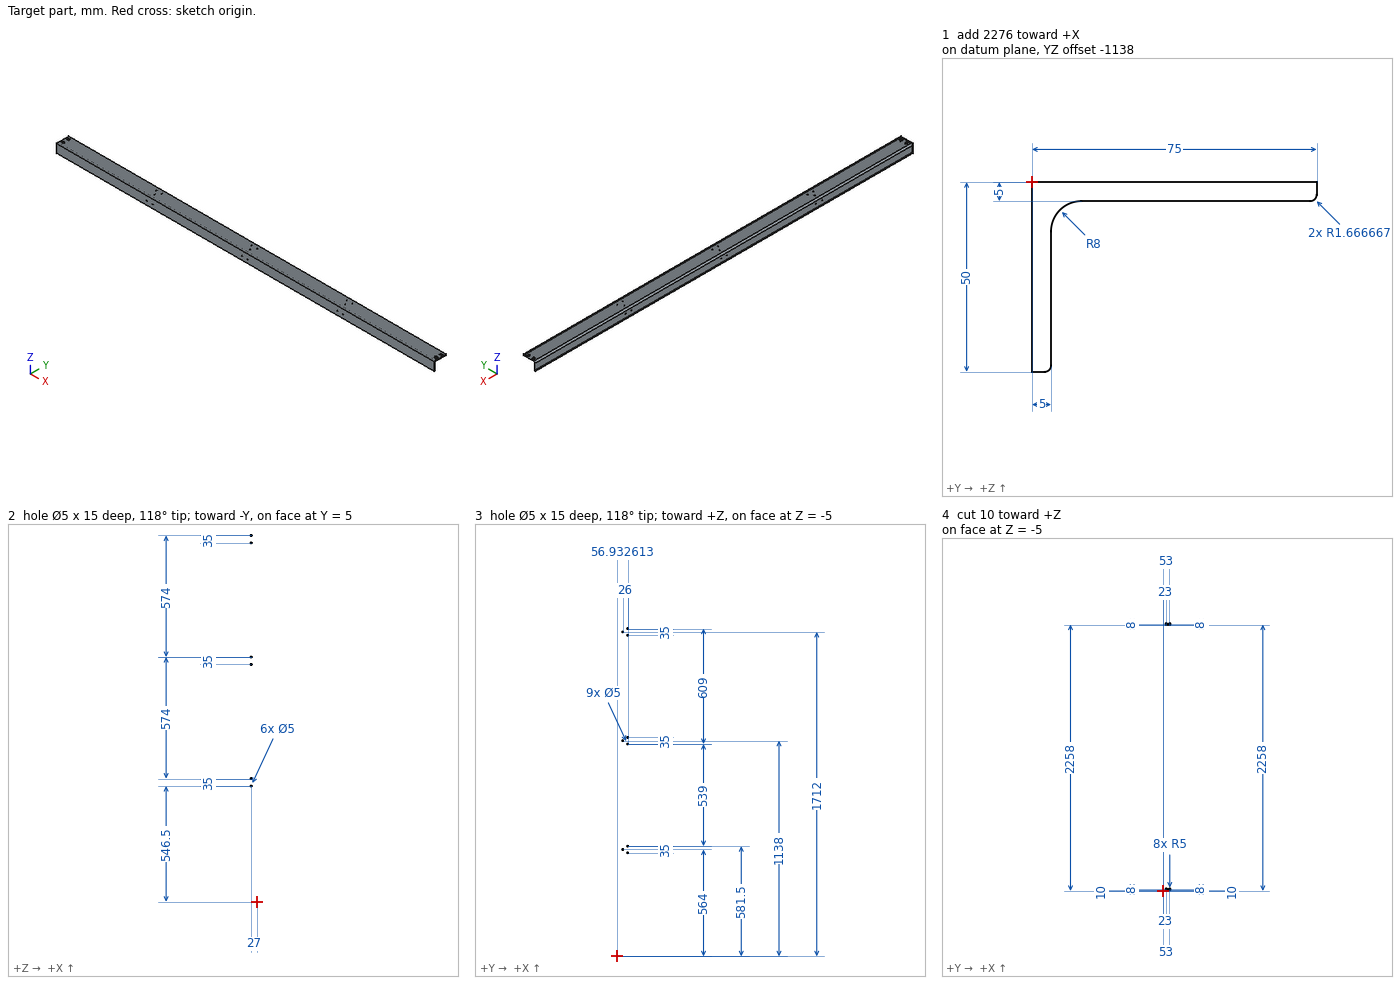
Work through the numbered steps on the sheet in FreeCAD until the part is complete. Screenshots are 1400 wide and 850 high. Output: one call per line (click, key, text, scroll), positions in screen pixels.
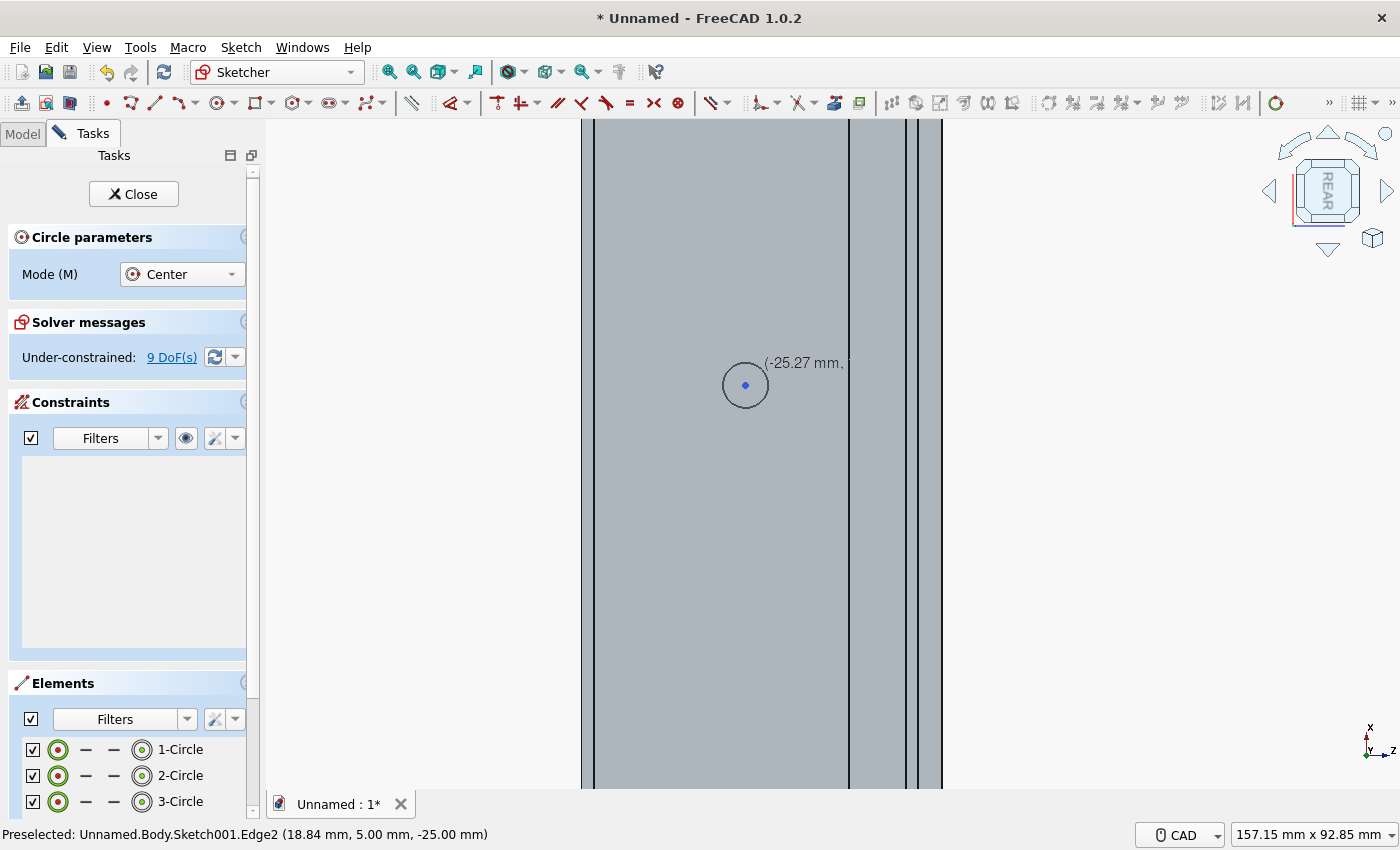
scroll(748, 632, up, 2)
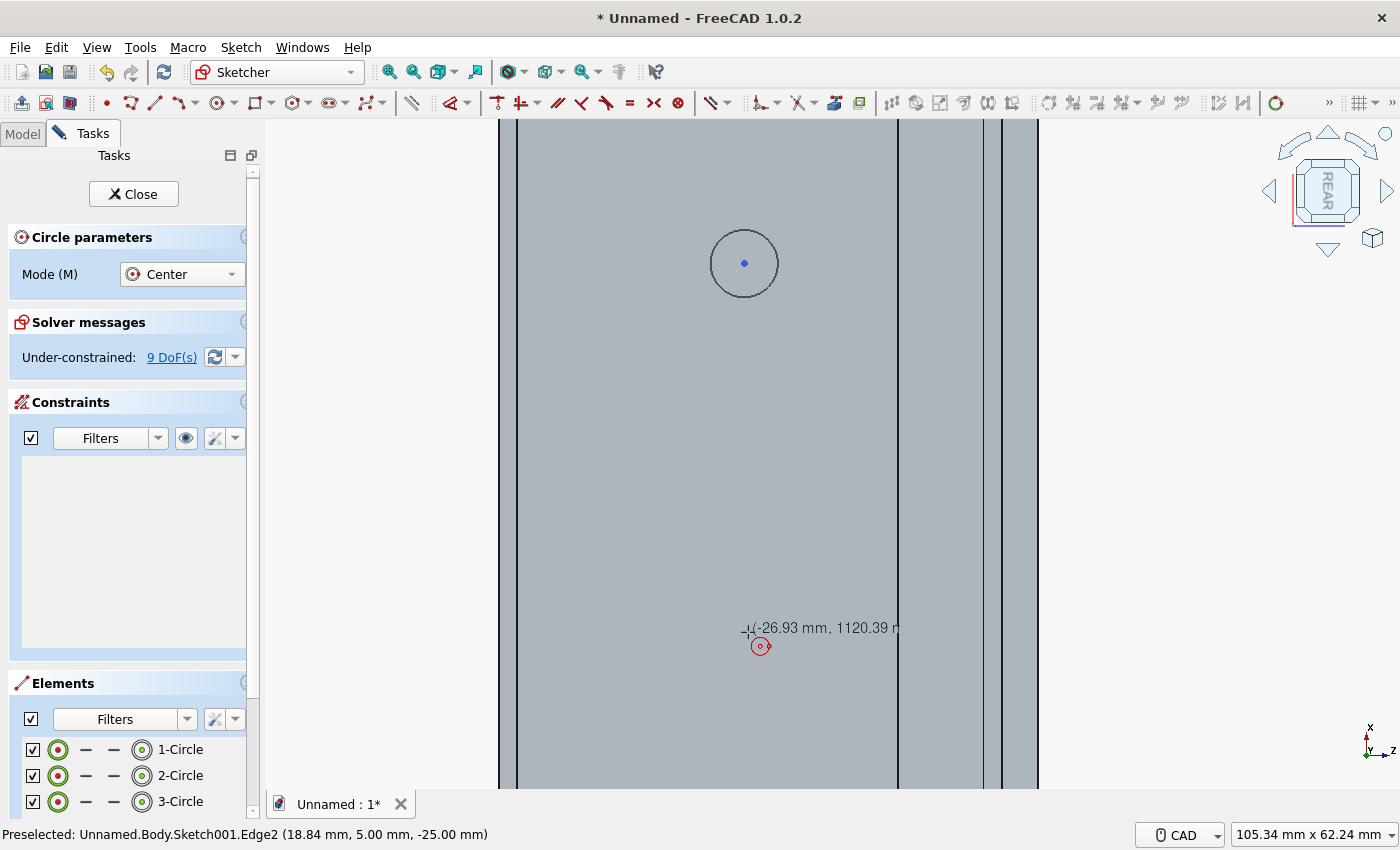
scroll(761, 372, down, 18)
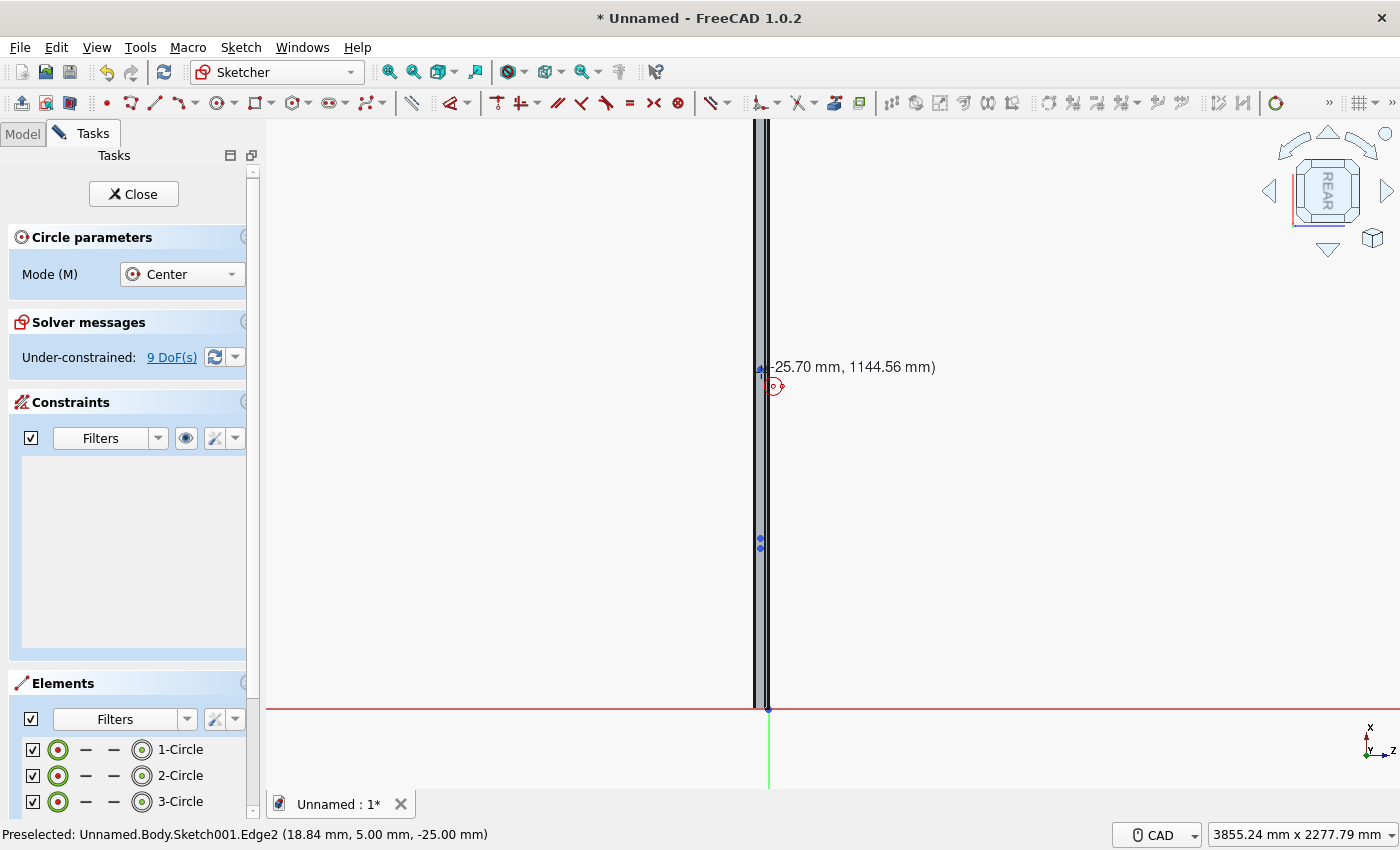
scroll(761, 379, up, 4)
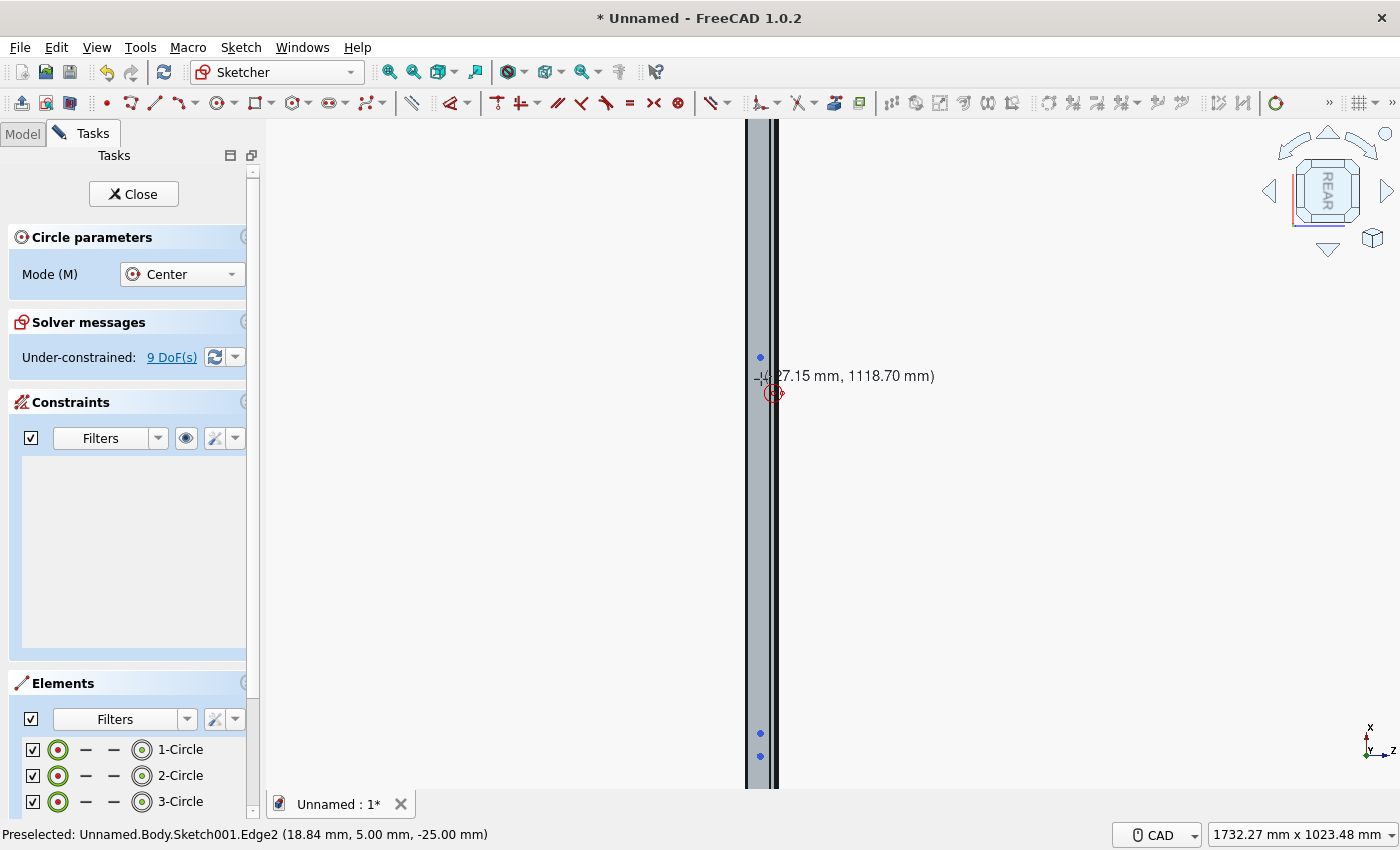
click(761, 380)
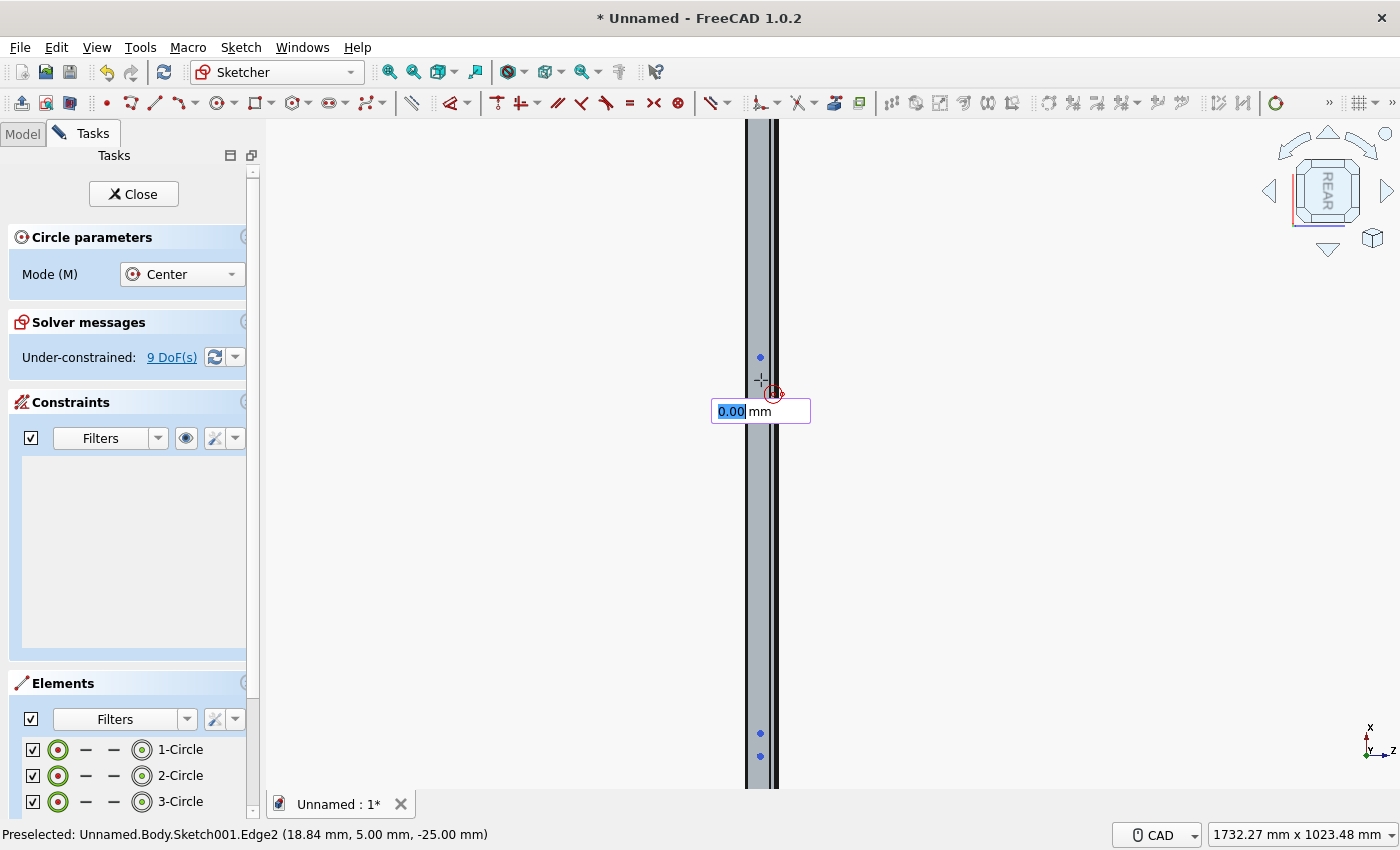
scroll(762, 378, up, 12)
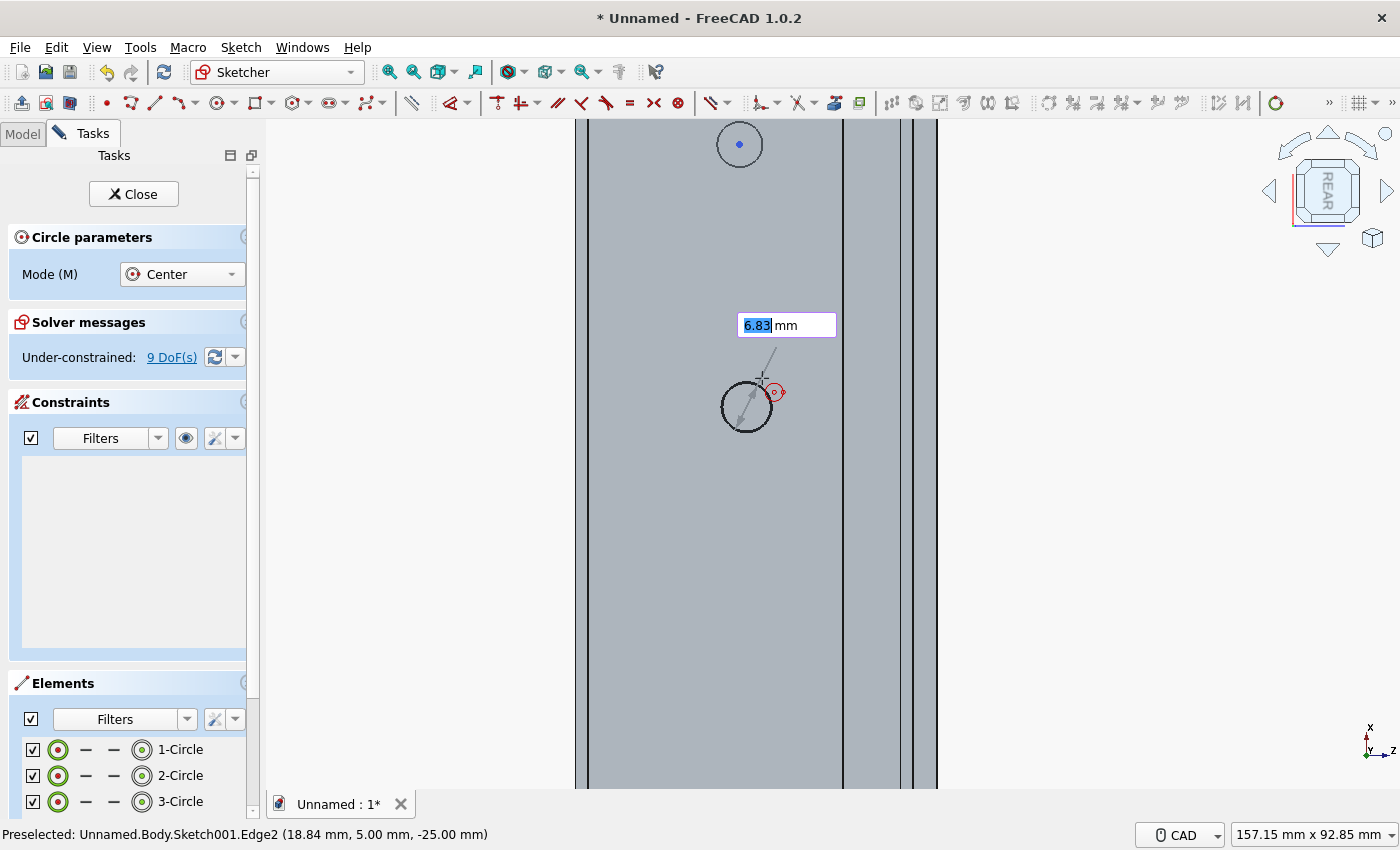
click(755, 379)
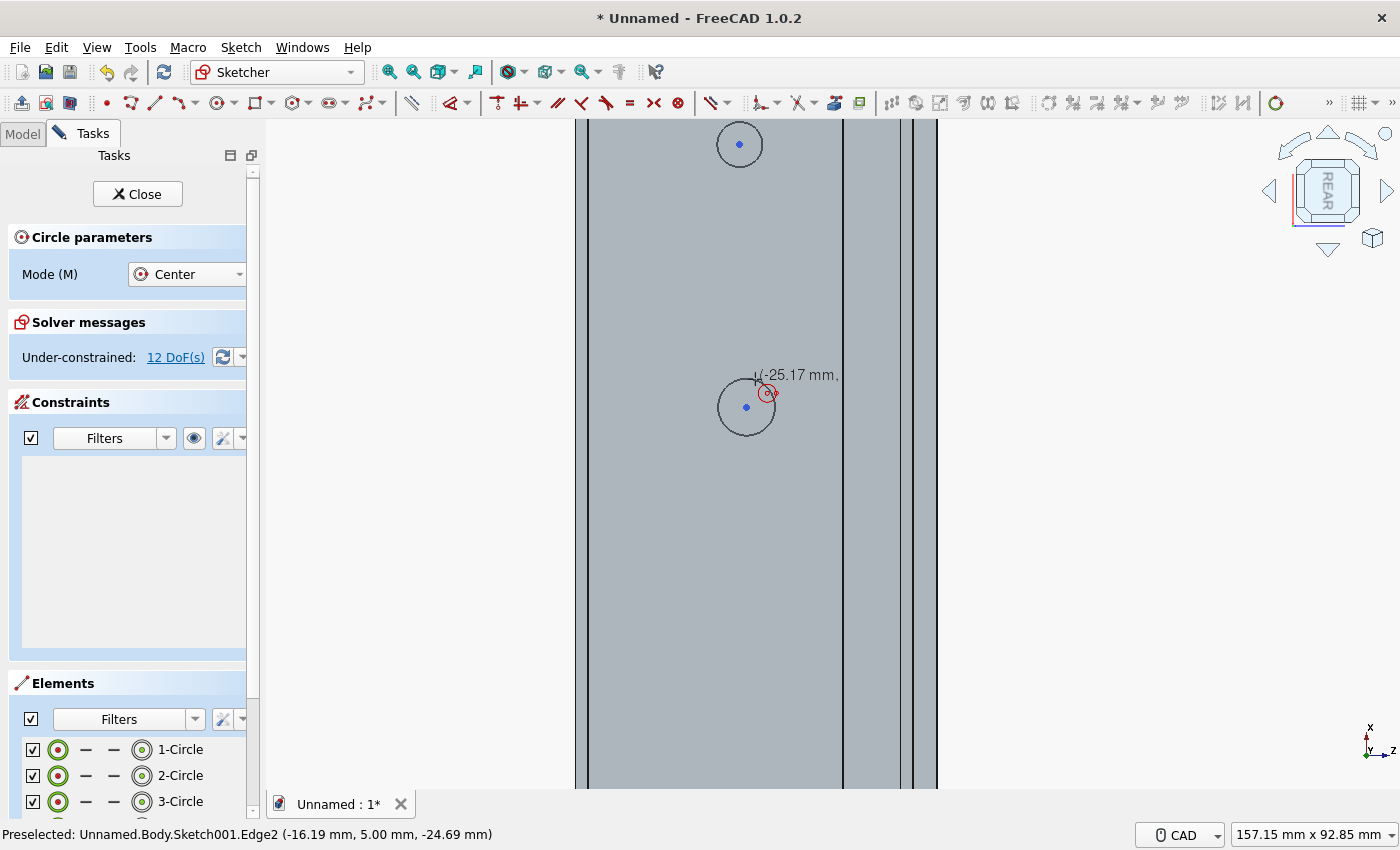
scroll(762, 379, down, 16)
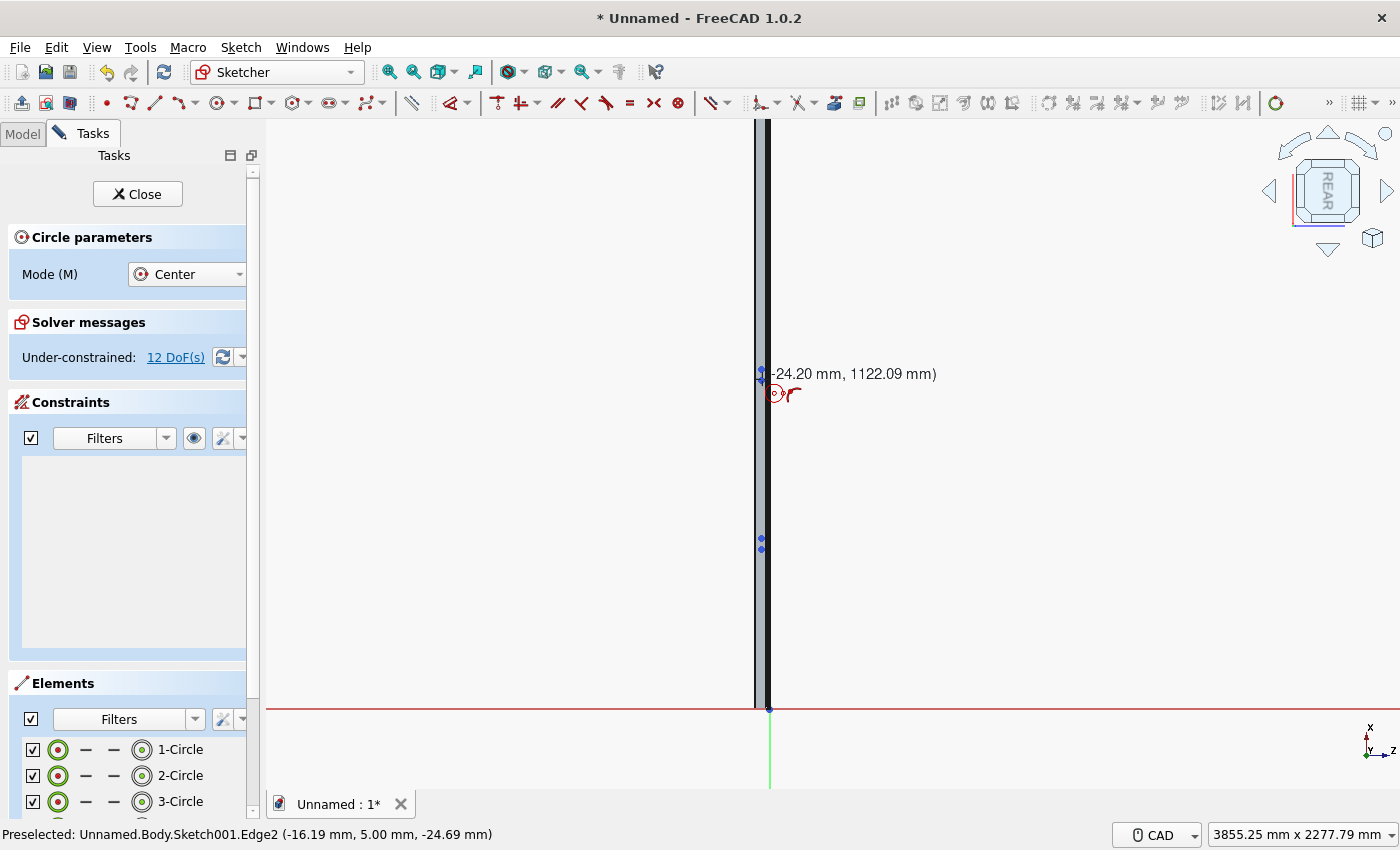
scroll(762, 201, up, 18)